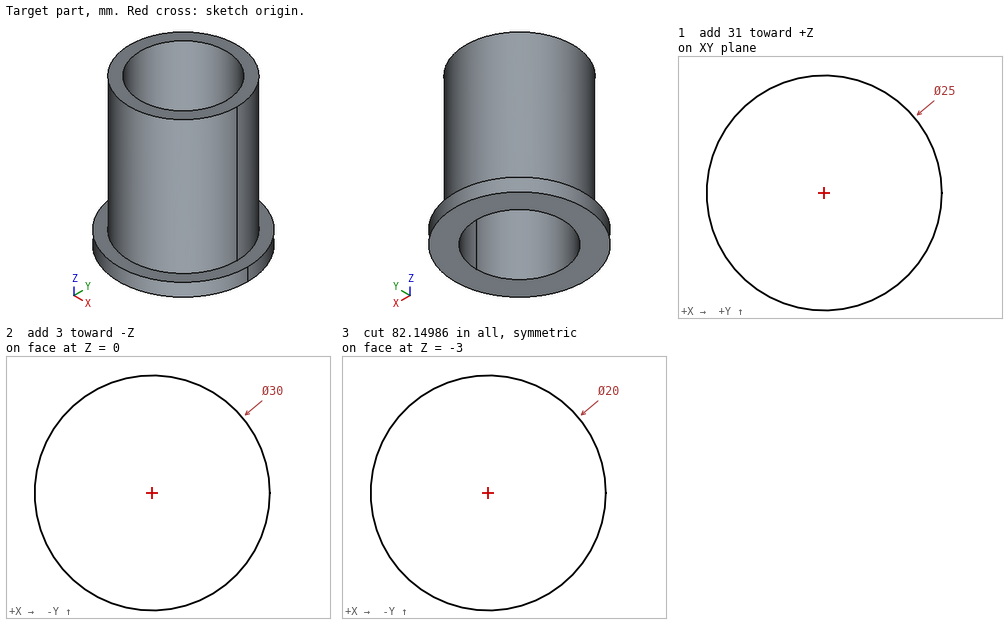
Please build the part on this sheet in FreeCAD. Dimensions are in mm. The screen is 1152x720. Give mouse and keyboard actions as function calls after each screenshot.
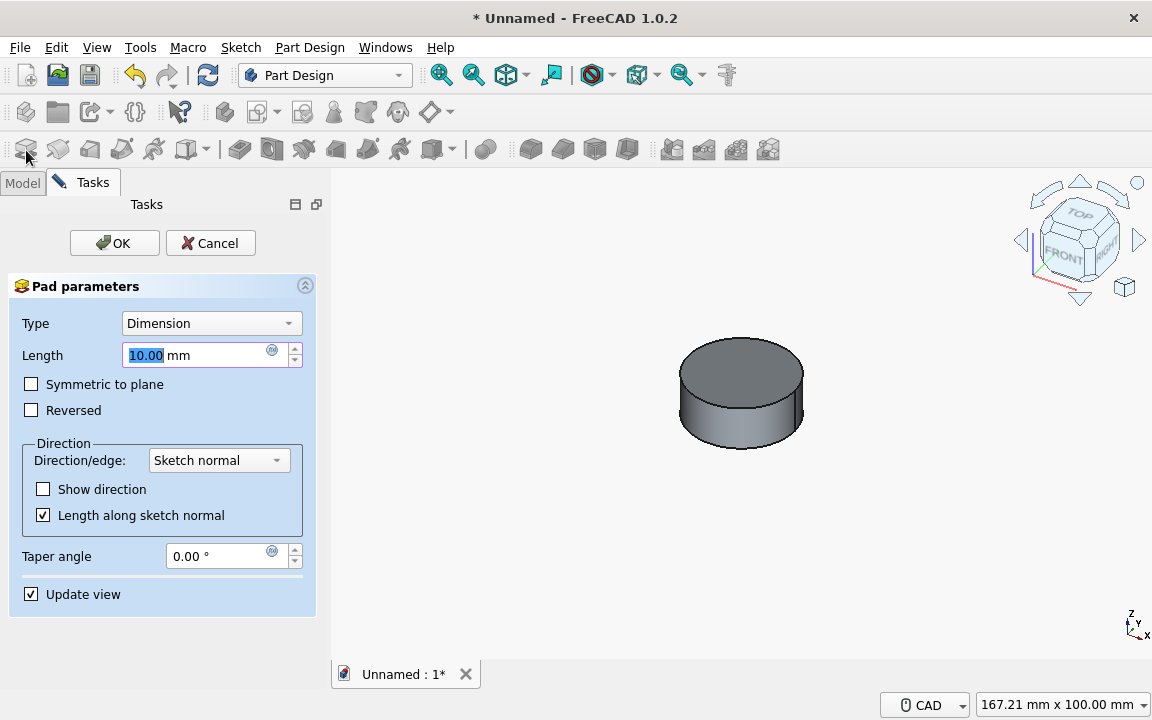
text(31)
key(Tab)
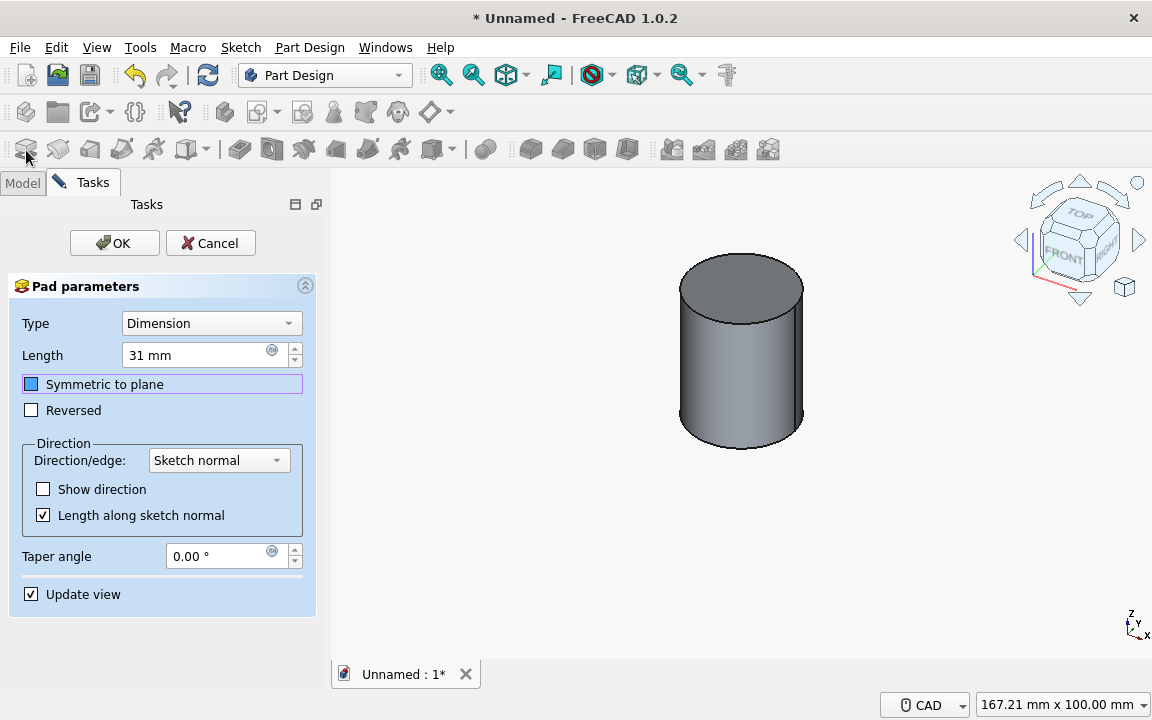
click(115, 243)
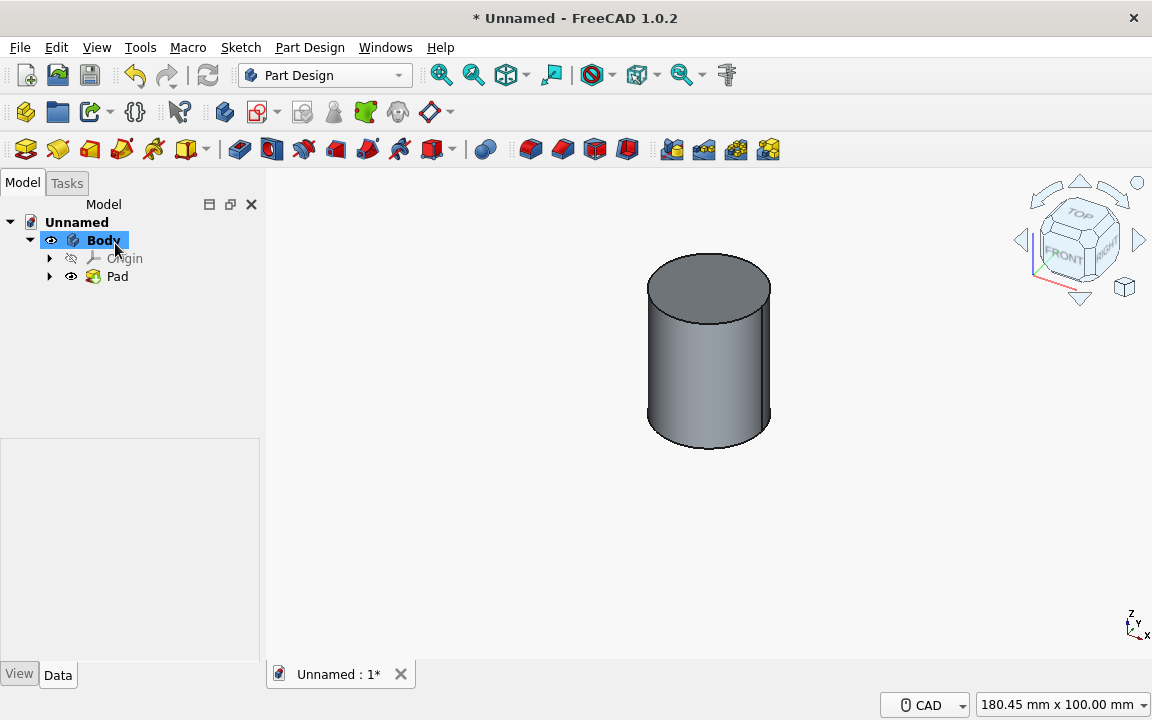
key(5)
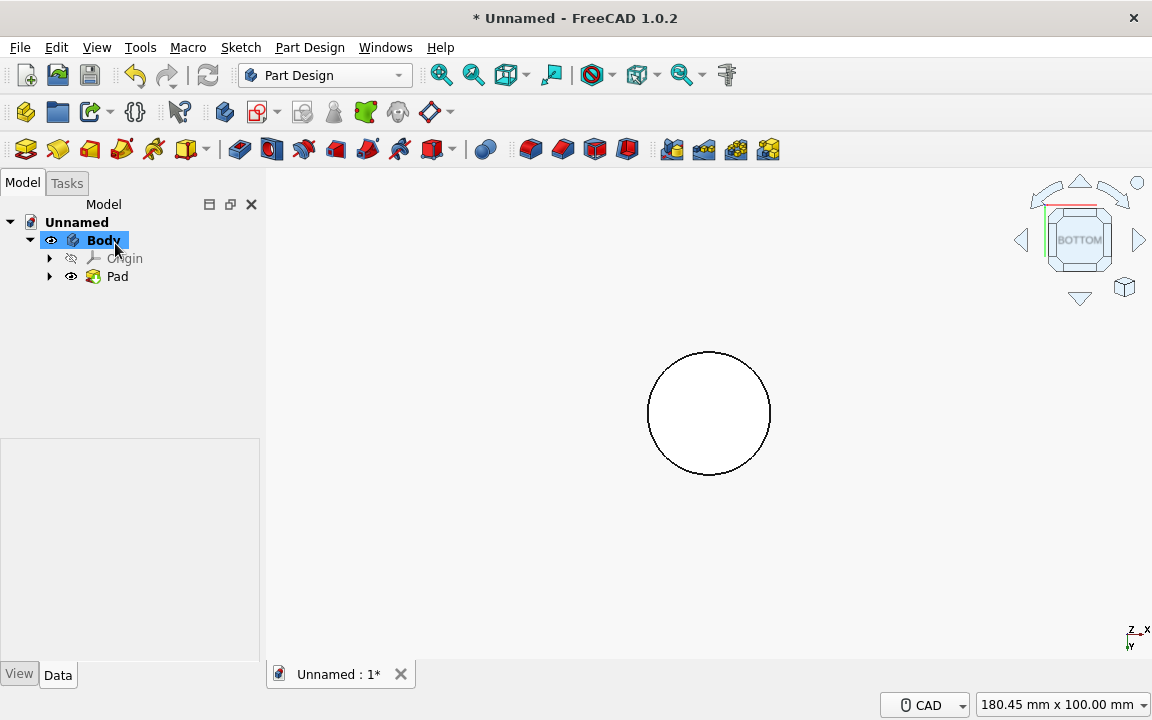
click(442, 76)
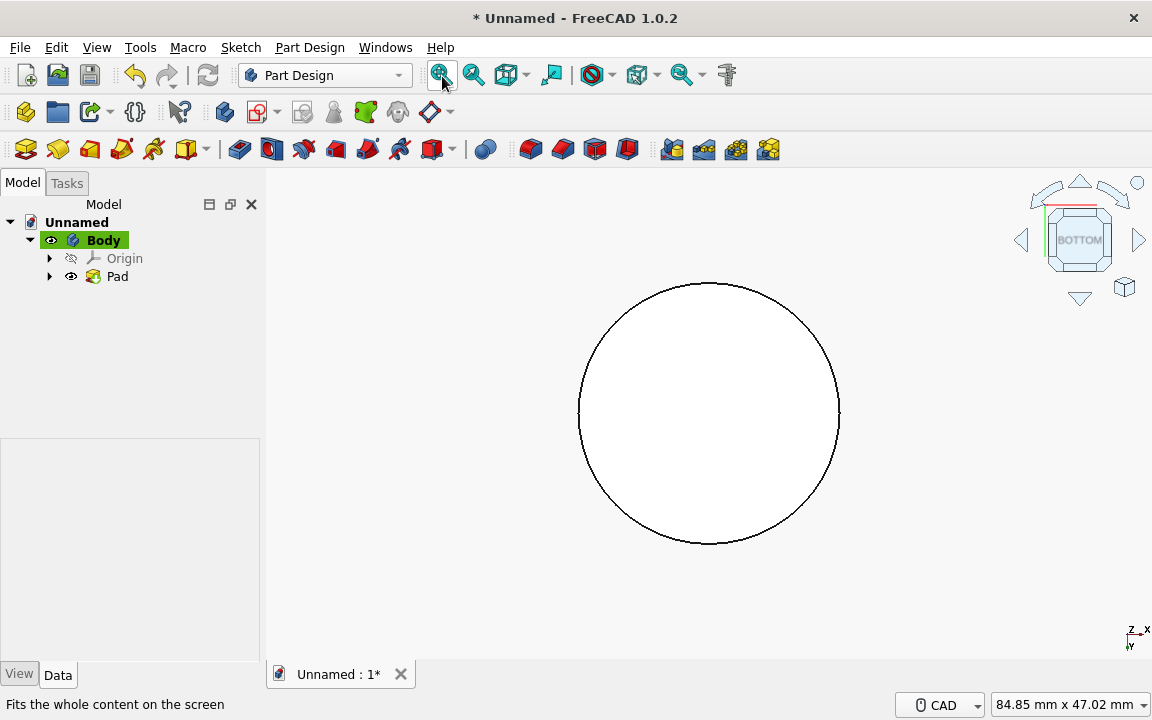
click(709, 412)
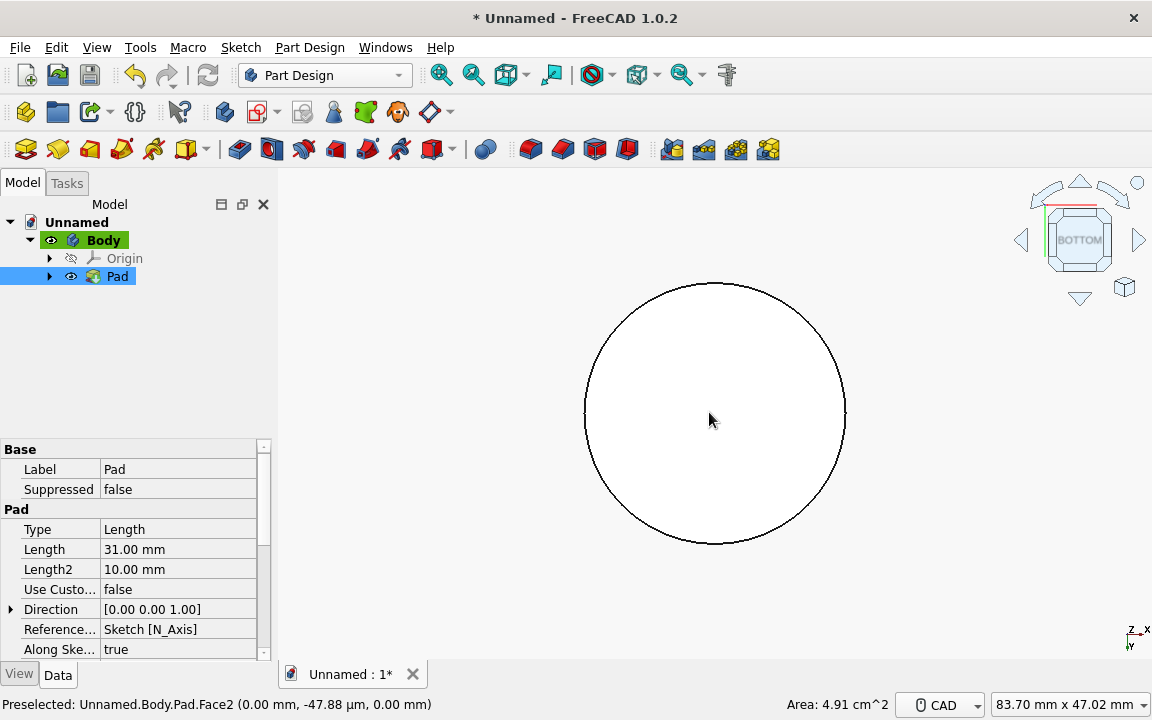
click(258, 112)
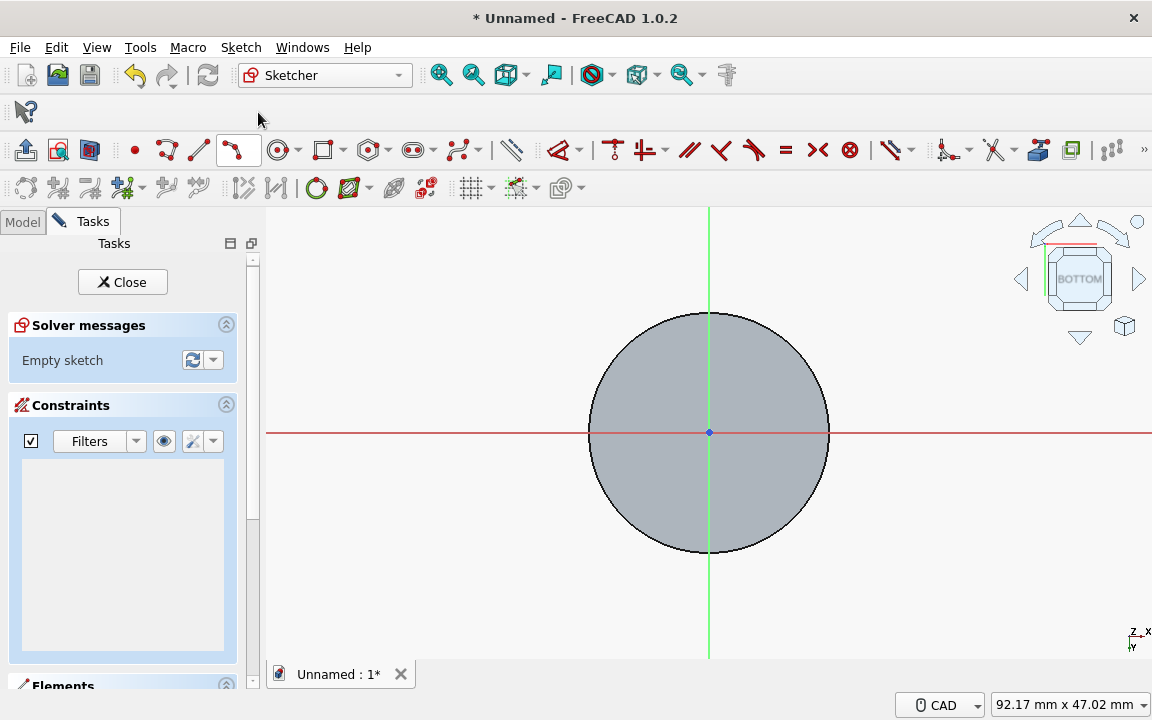
click(278, 150)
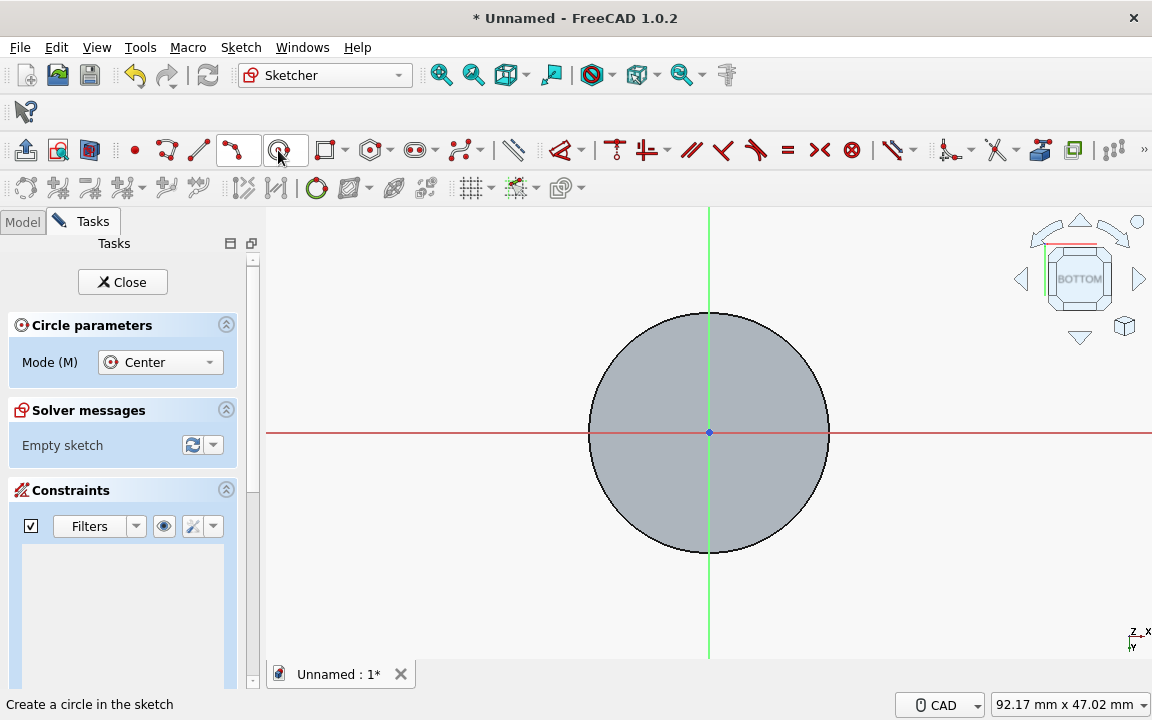
click(709, 433)
click(811, 331)
key(Escape)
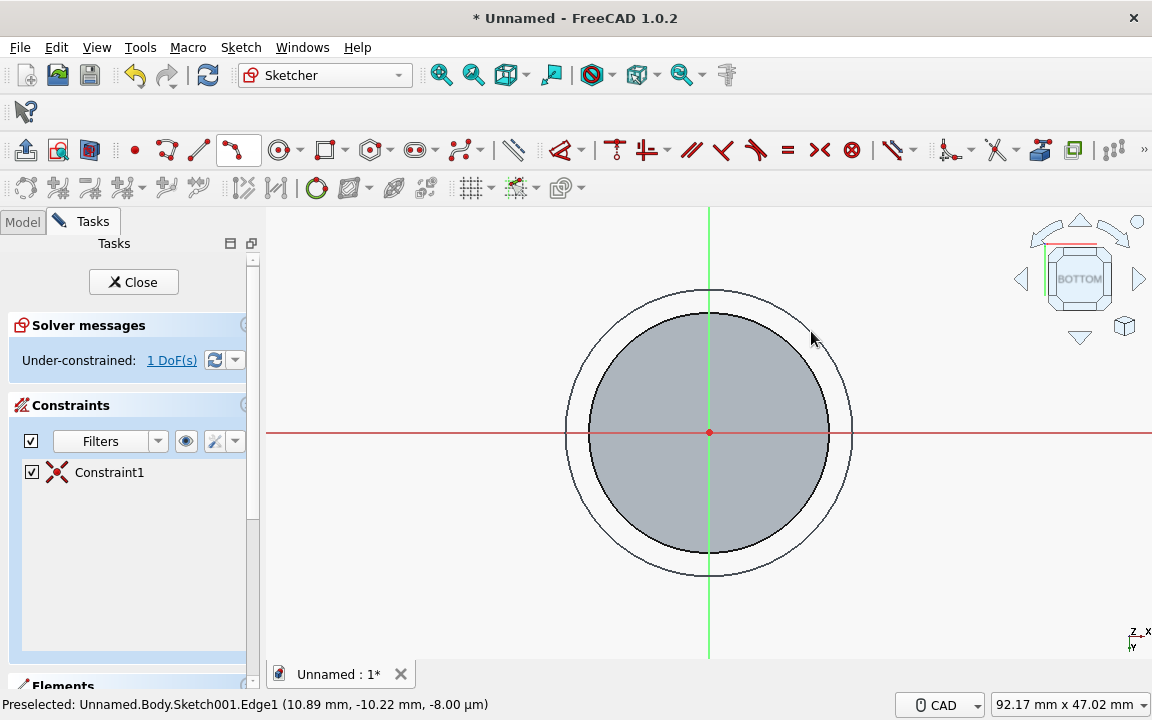
click(560, 150)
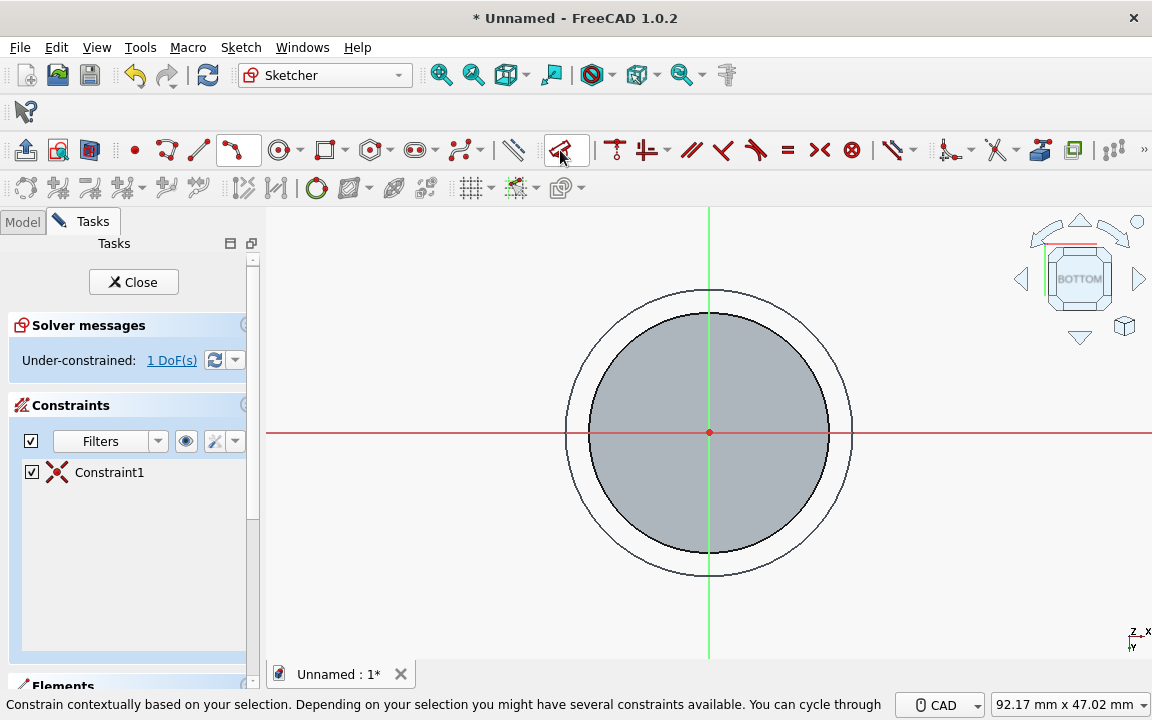
click(810, 331)
click(833, 308)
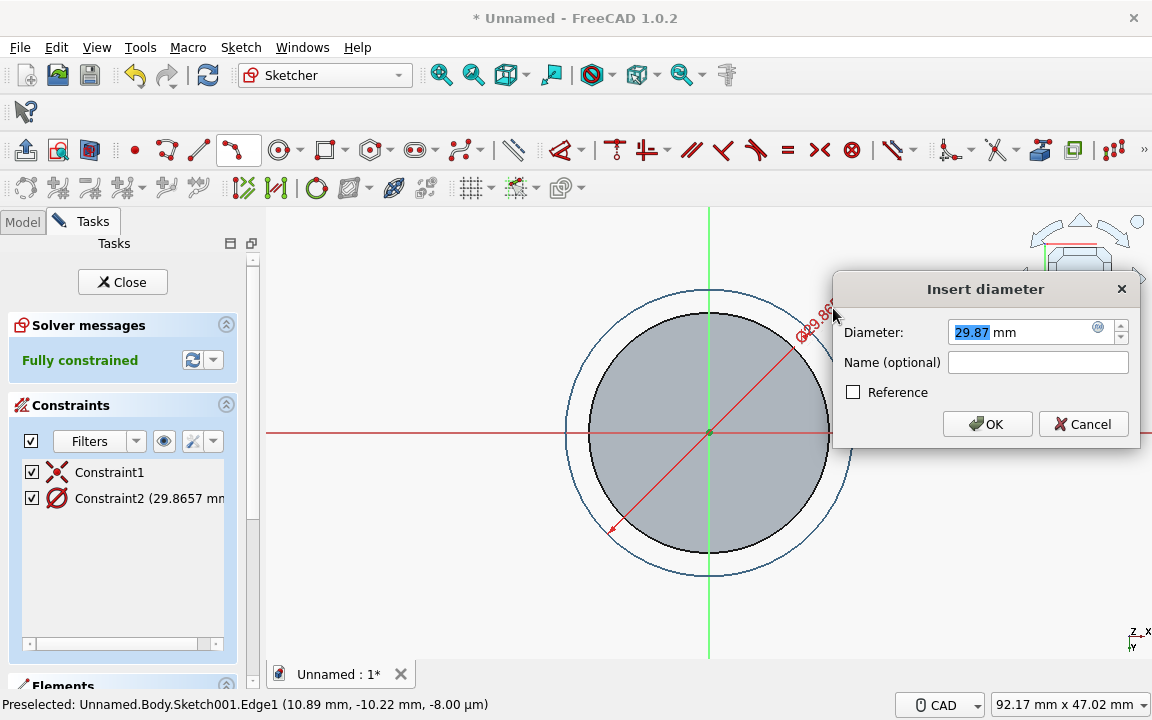
text(30)
key(Return)
key(Escape)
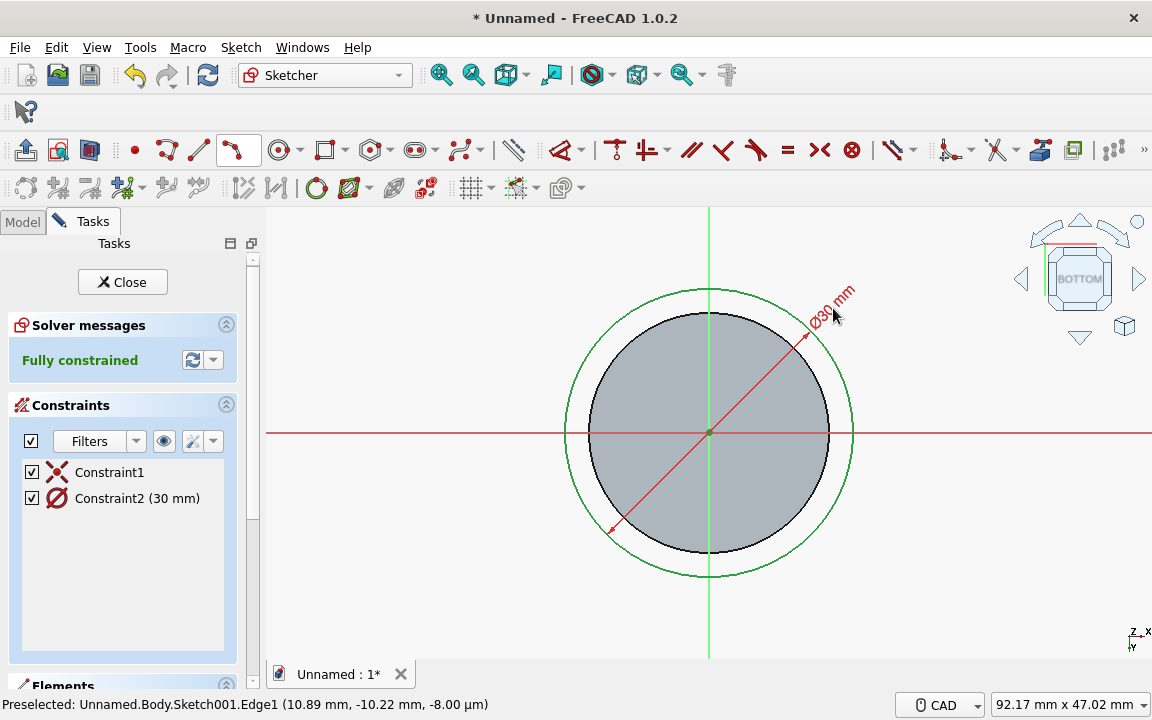
click(123, 282)